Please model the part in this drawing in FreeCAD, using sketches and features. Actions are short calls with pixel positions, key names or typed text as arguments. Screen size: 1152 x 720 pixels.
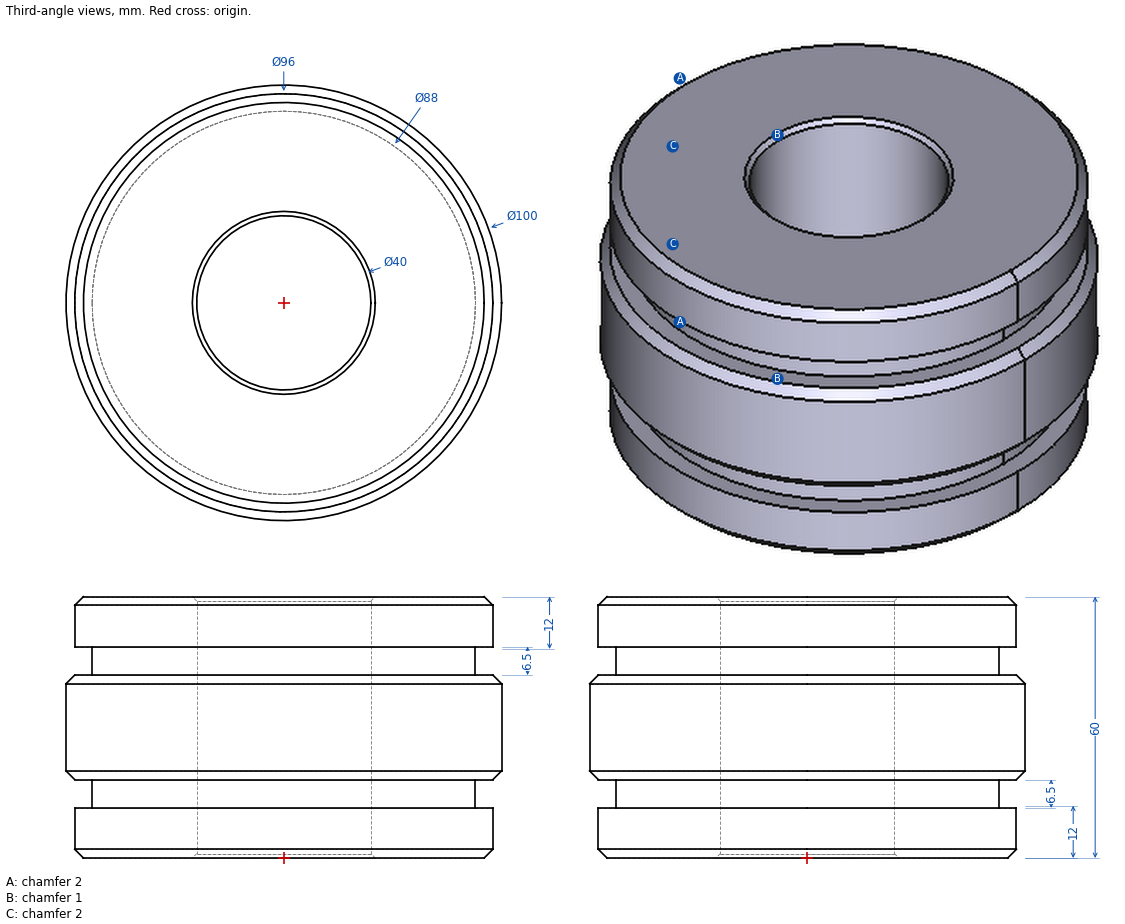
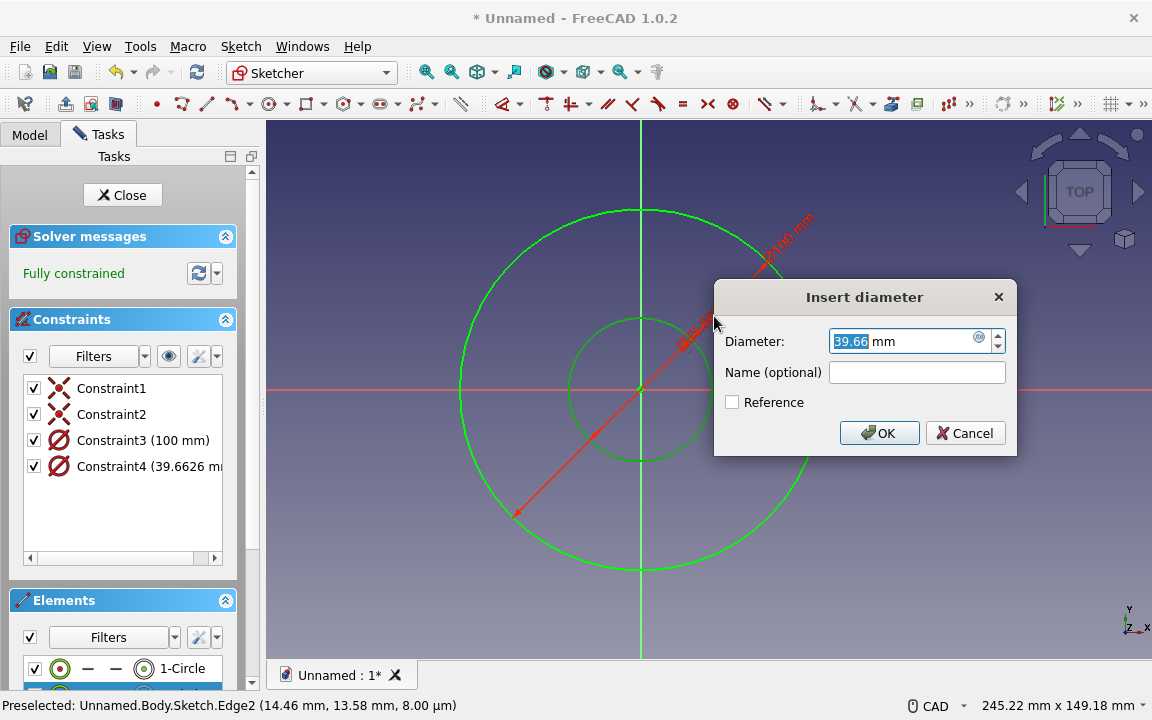
text(40)
key(Return)
key(Escape)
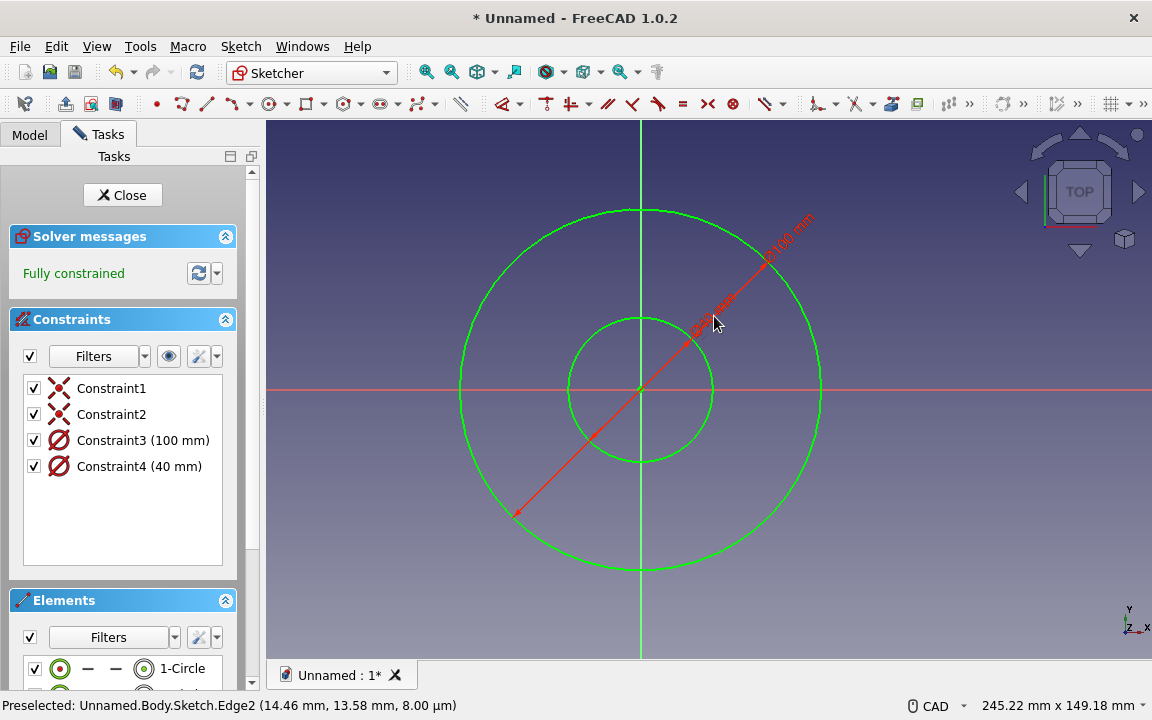
click(123, 195)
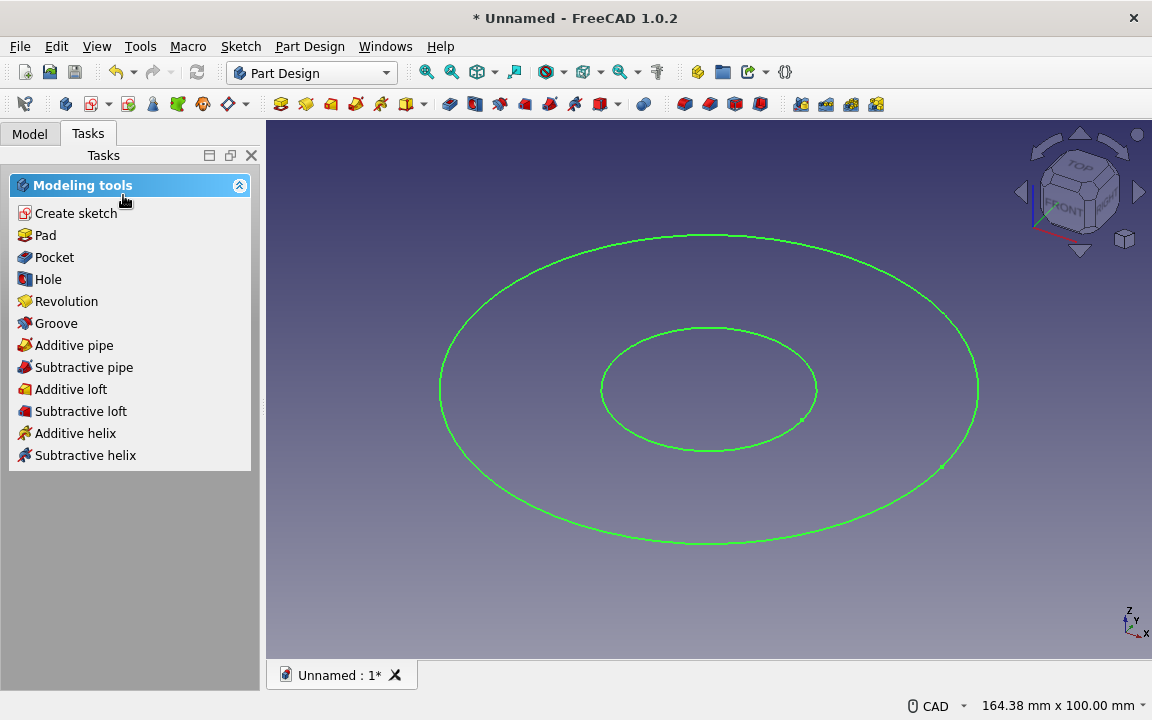
click(281, 104)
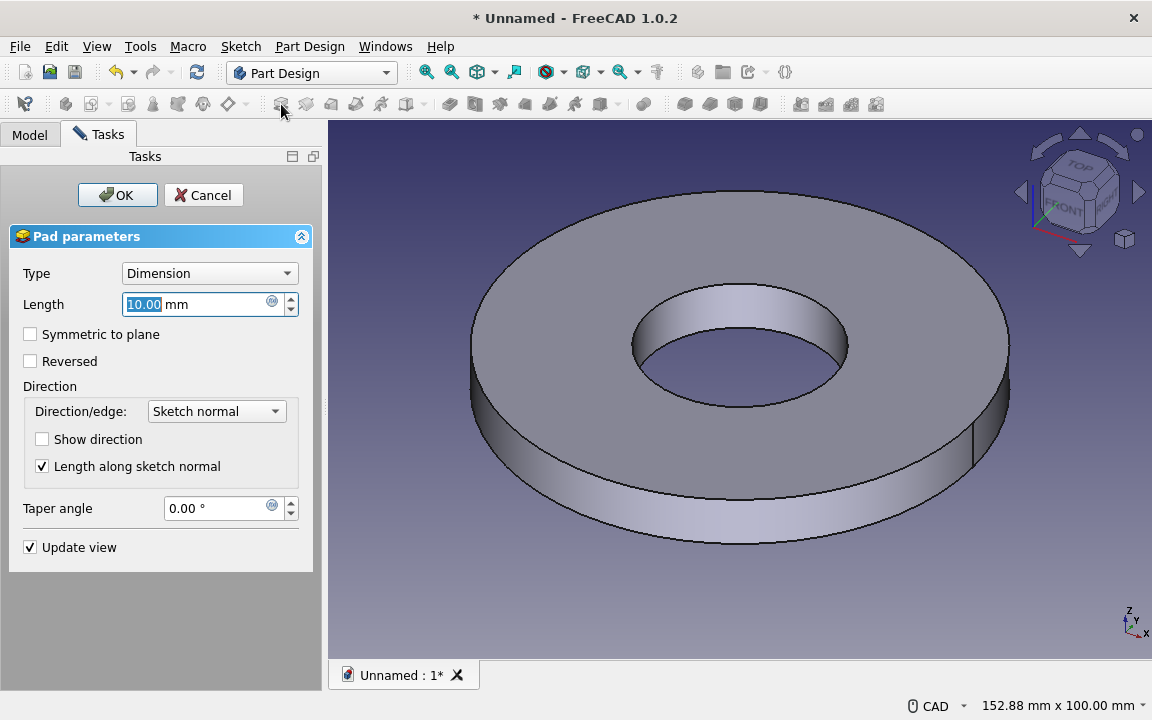
text(60)
key(Tab)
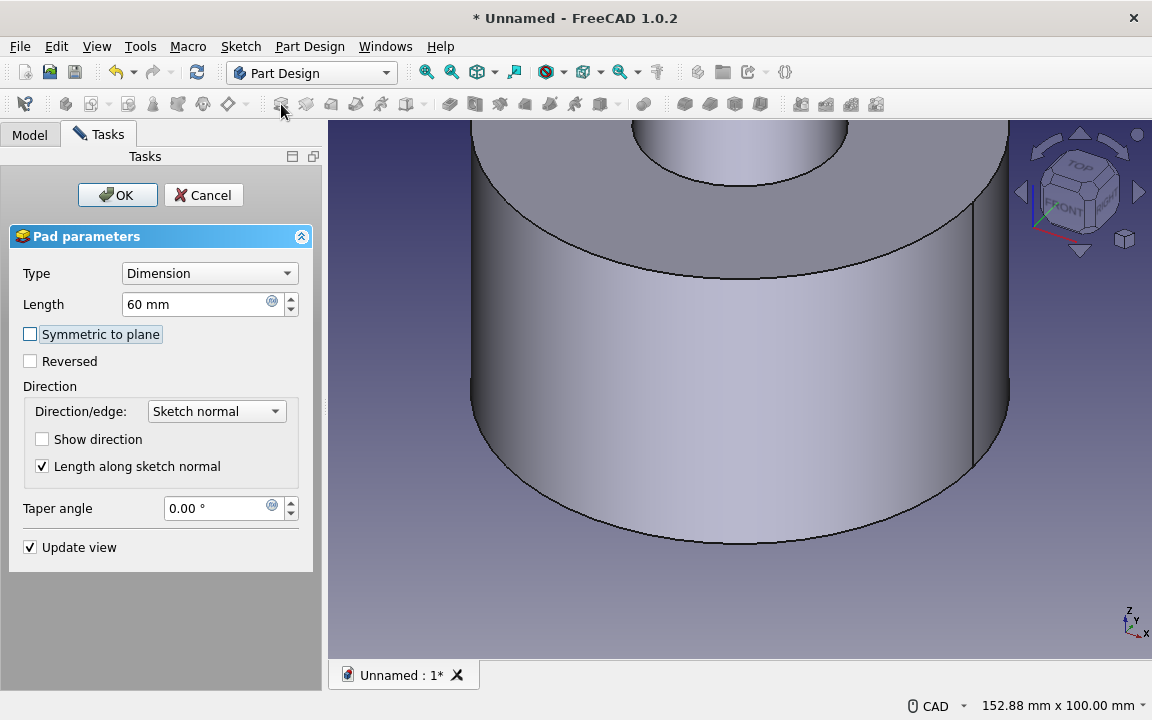
click(118, 195)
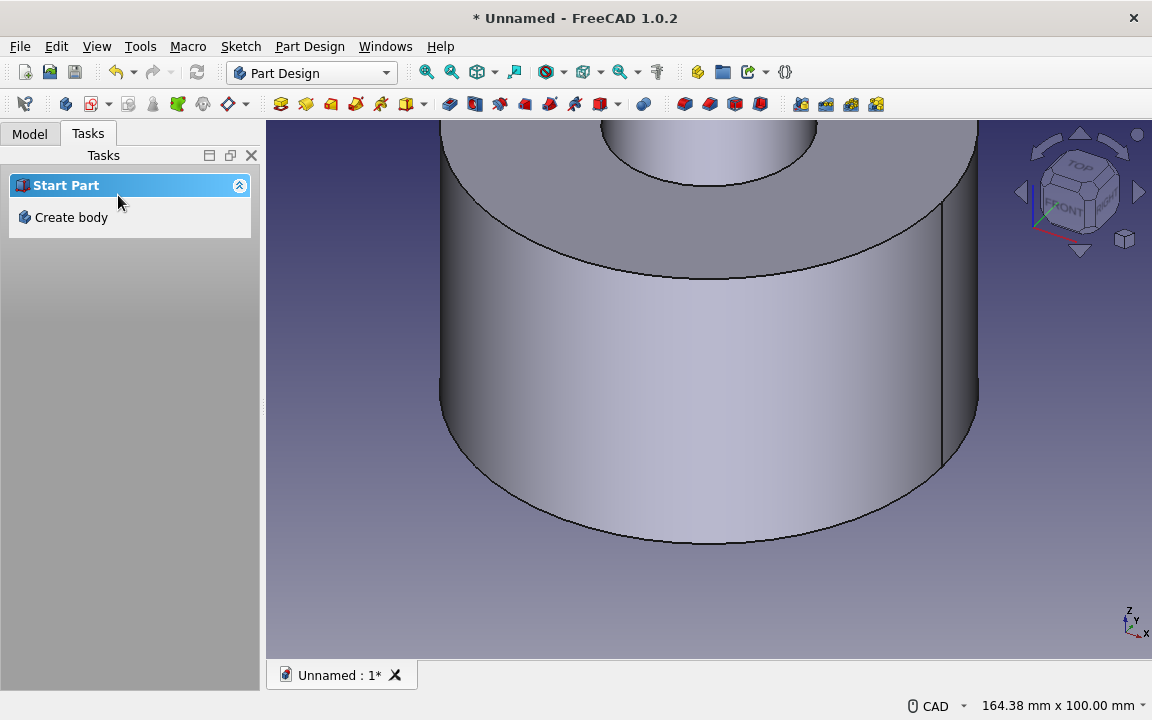
click(427, 72)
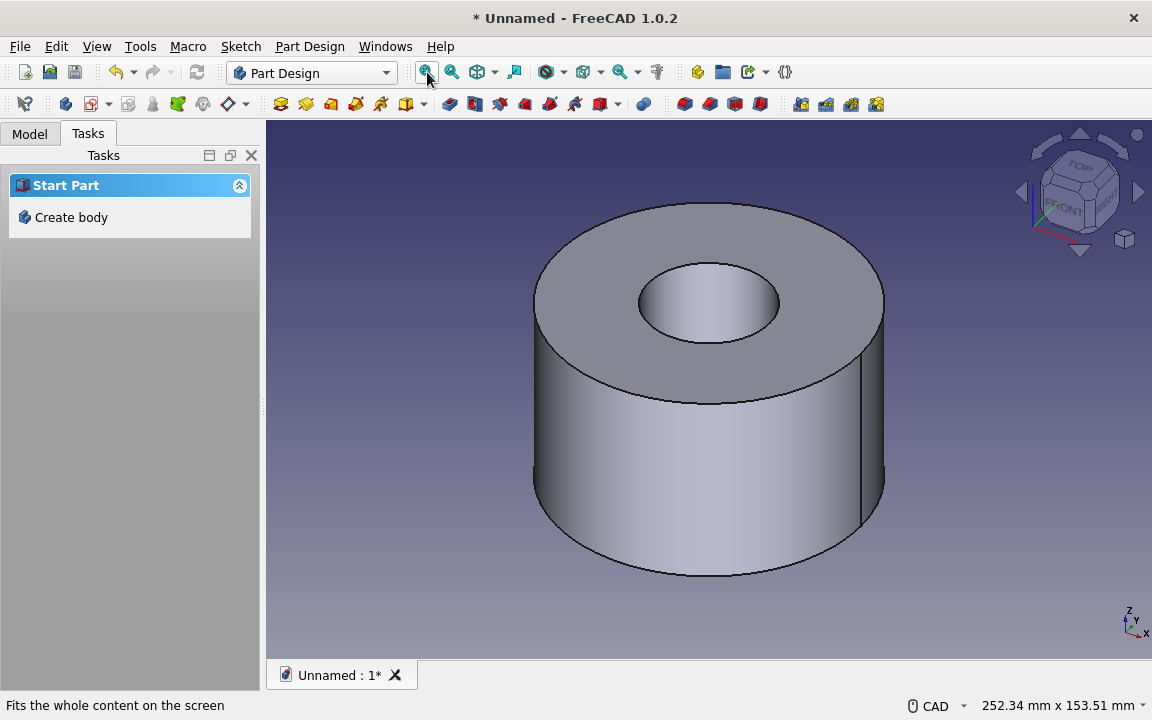
click(30, 134)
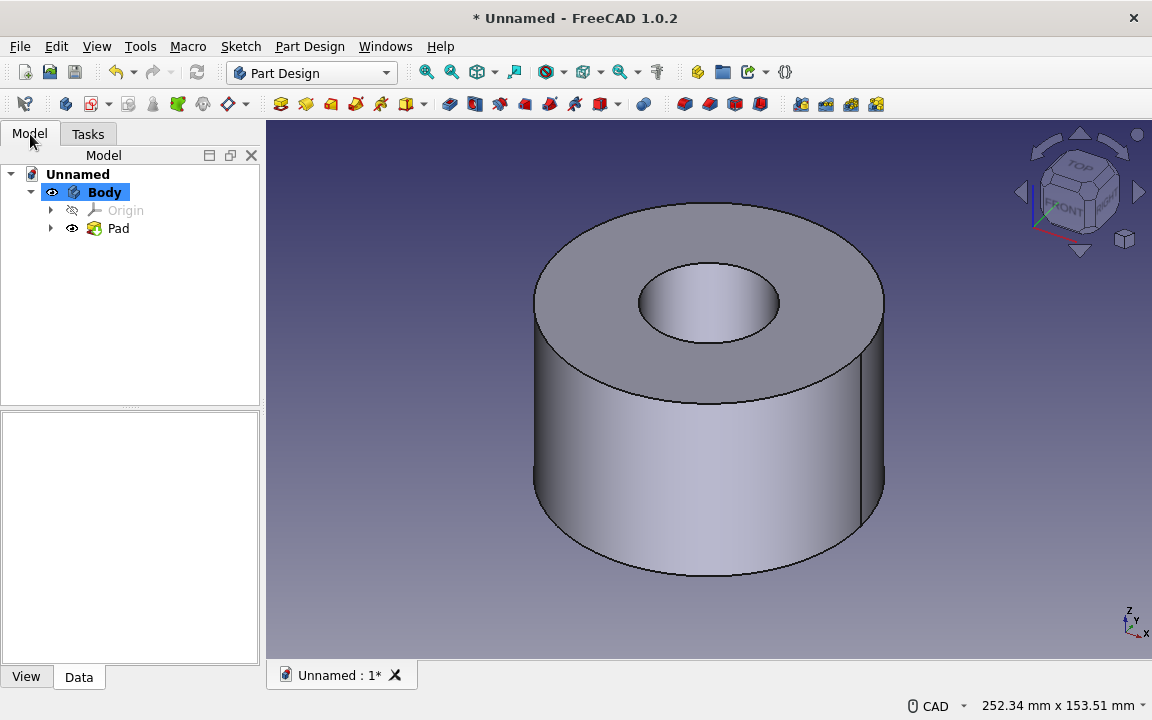
click(51, 210)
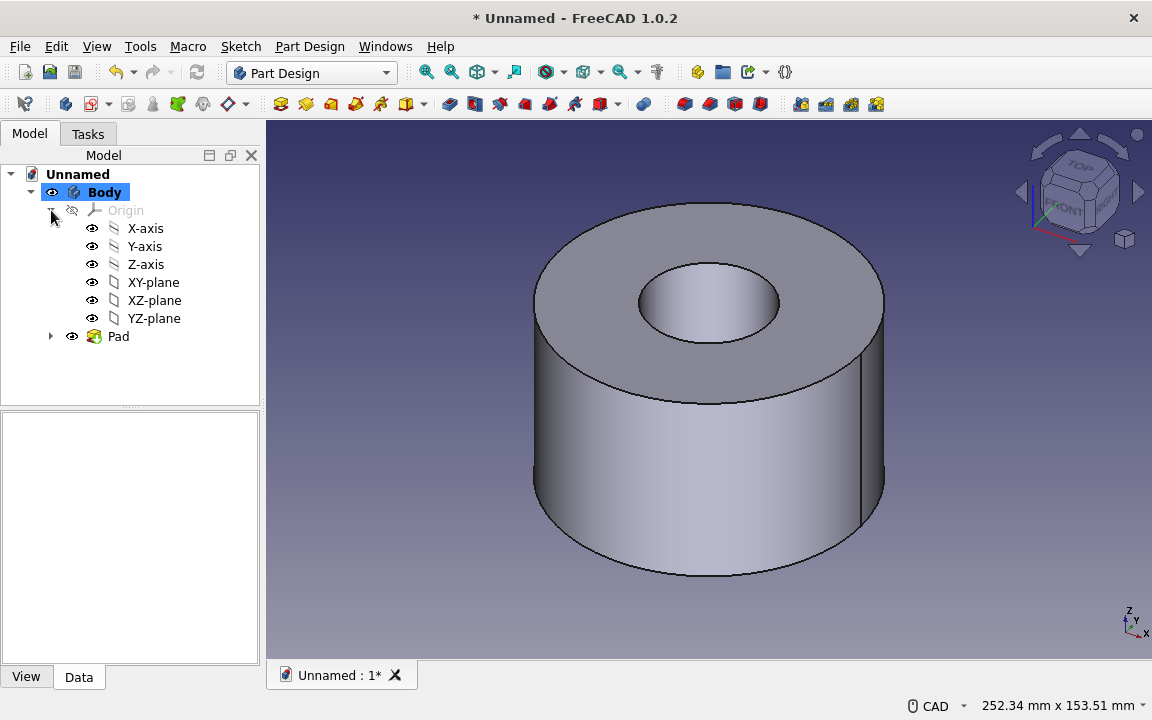
click(137, 282)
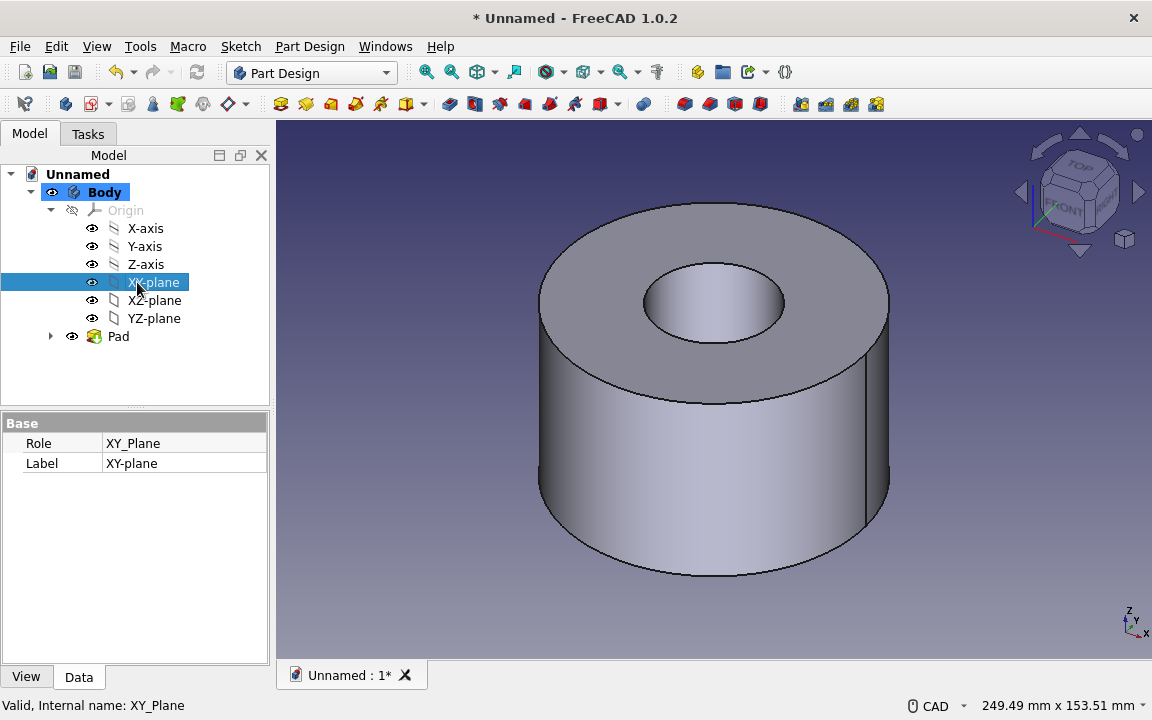
click(228, 104)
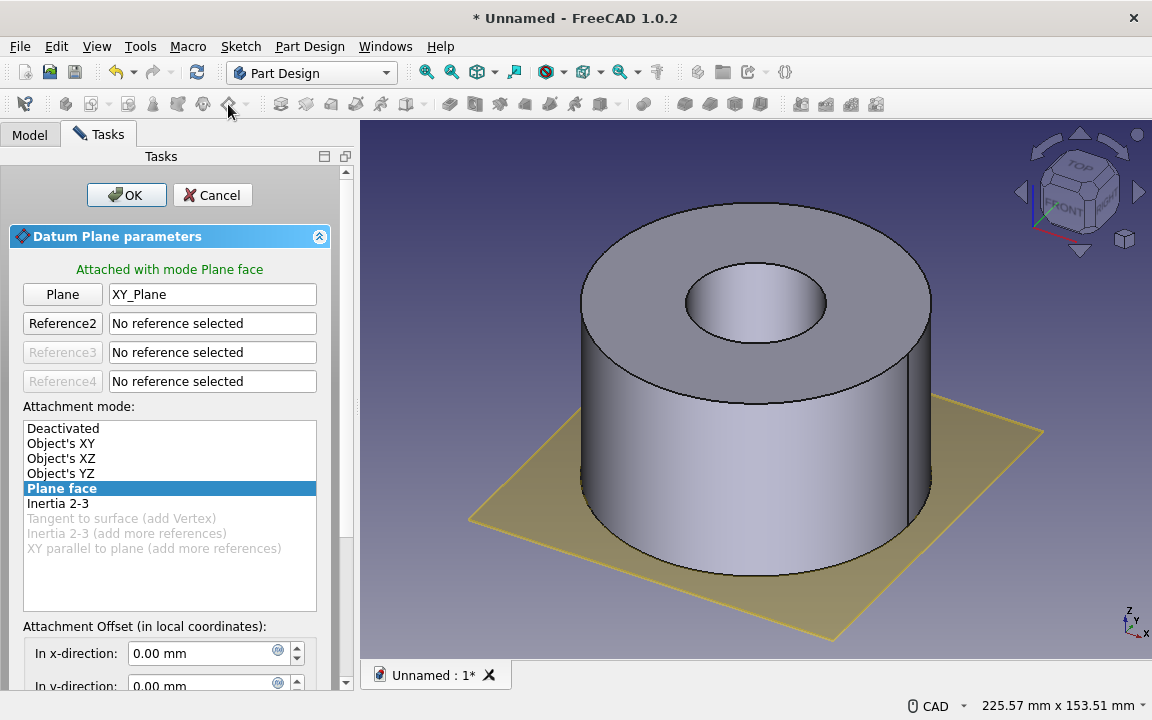
scroll(346, 428, down, 2)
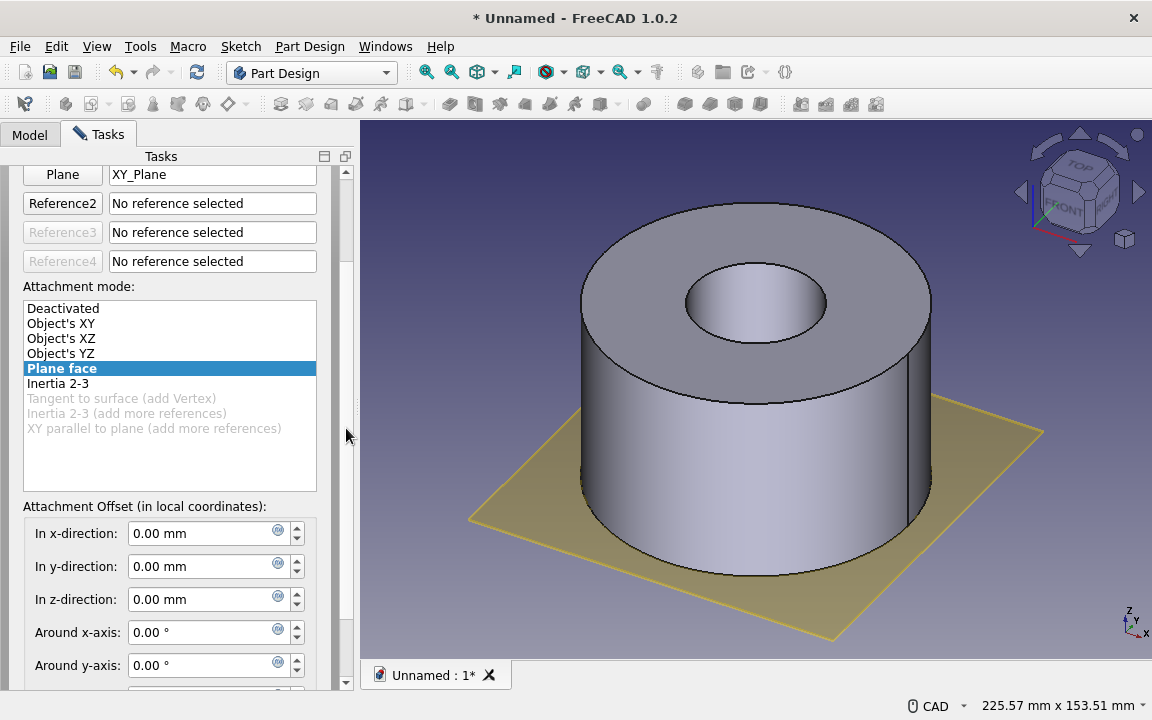
triple_click(210, 600)